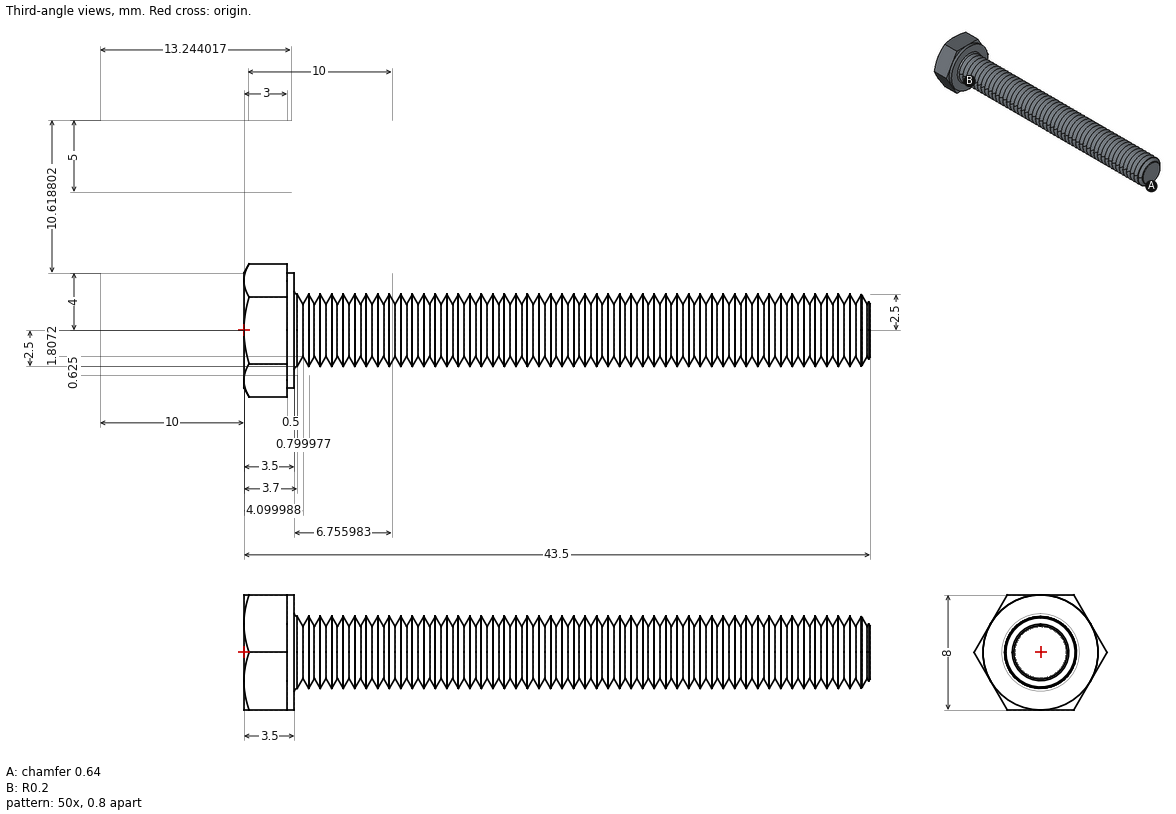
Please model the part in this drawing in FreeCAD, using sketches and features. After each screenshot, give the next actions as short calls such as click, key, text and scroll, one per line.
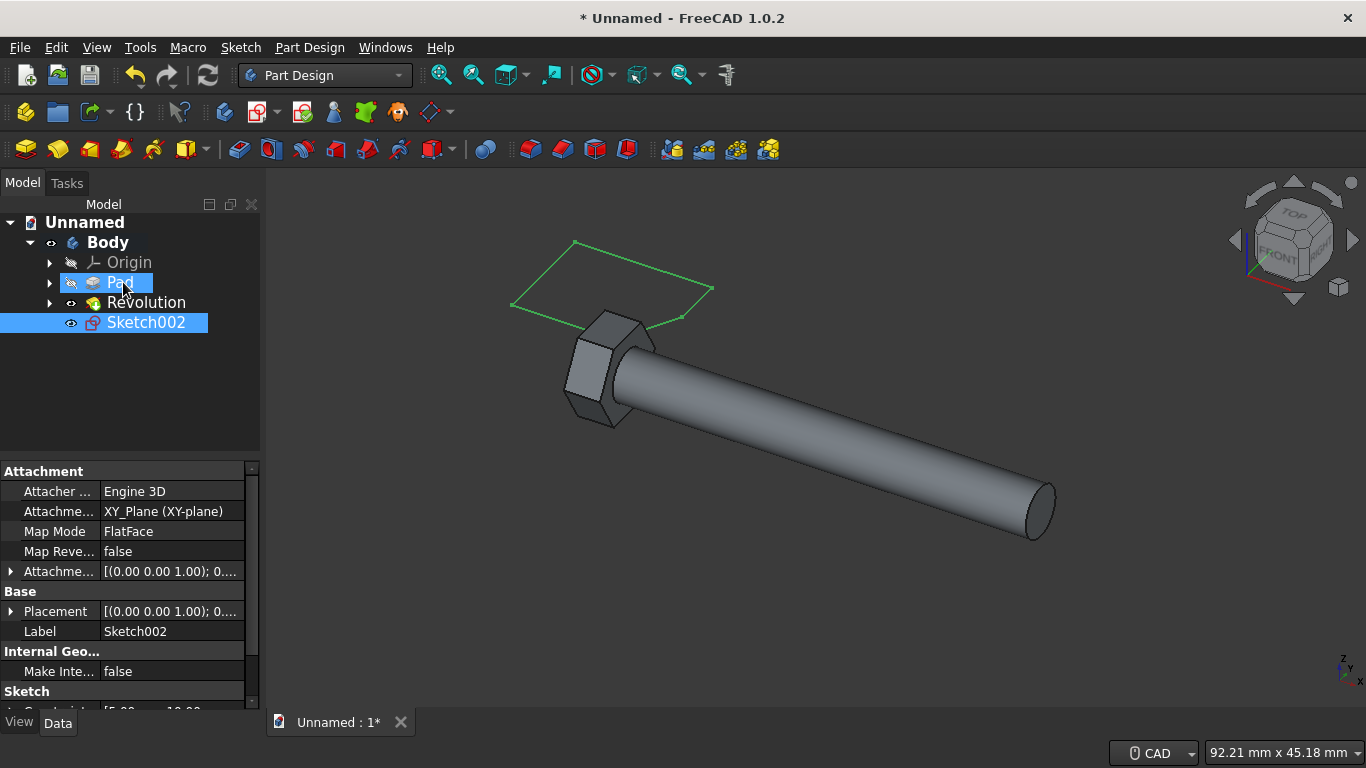
click(304, 150)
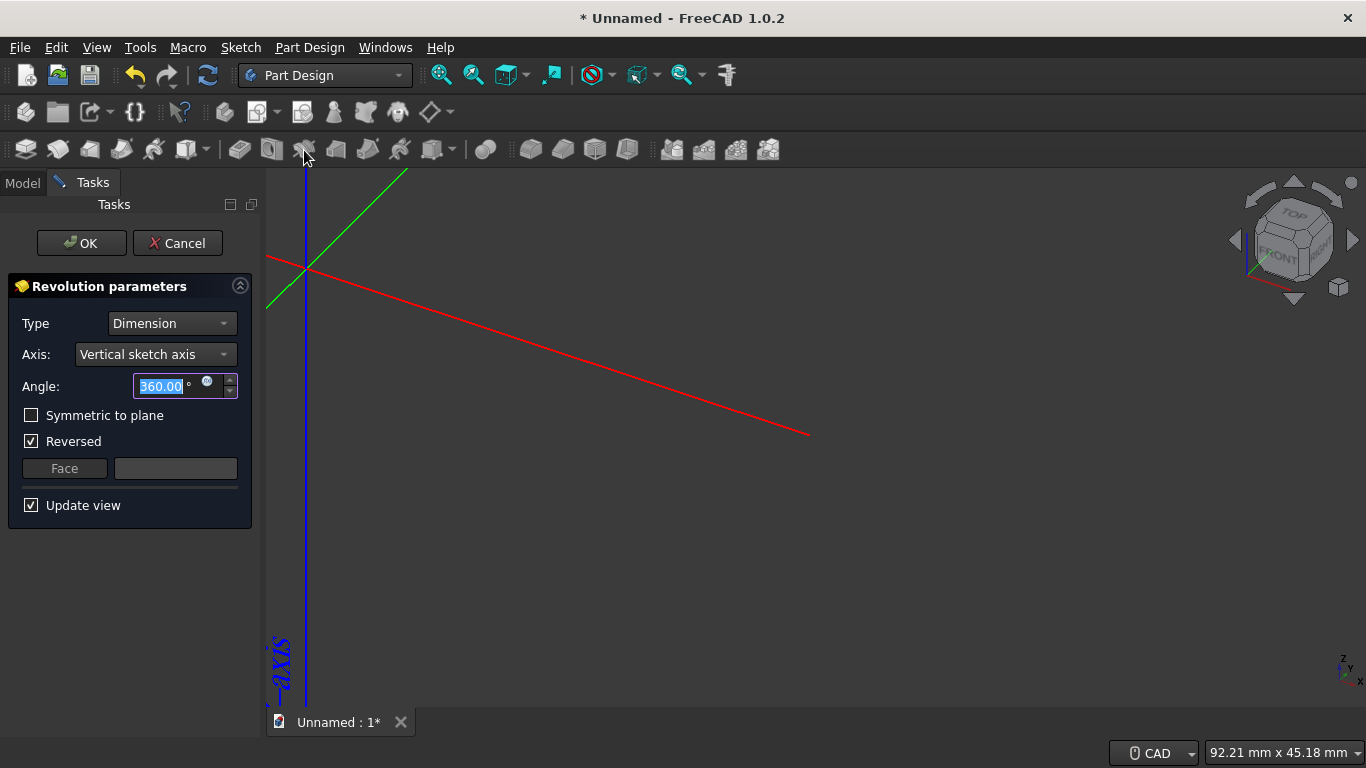
click(156, 354)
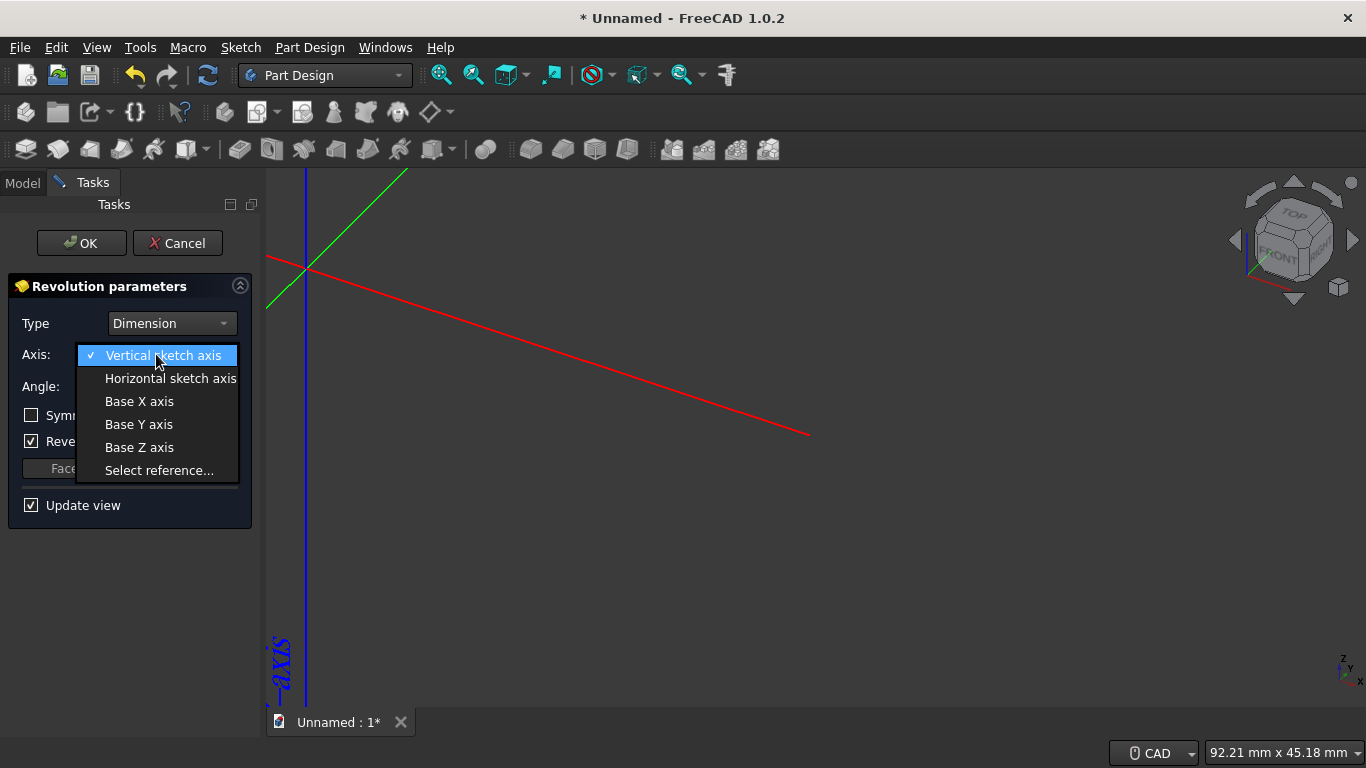
click(156, 378)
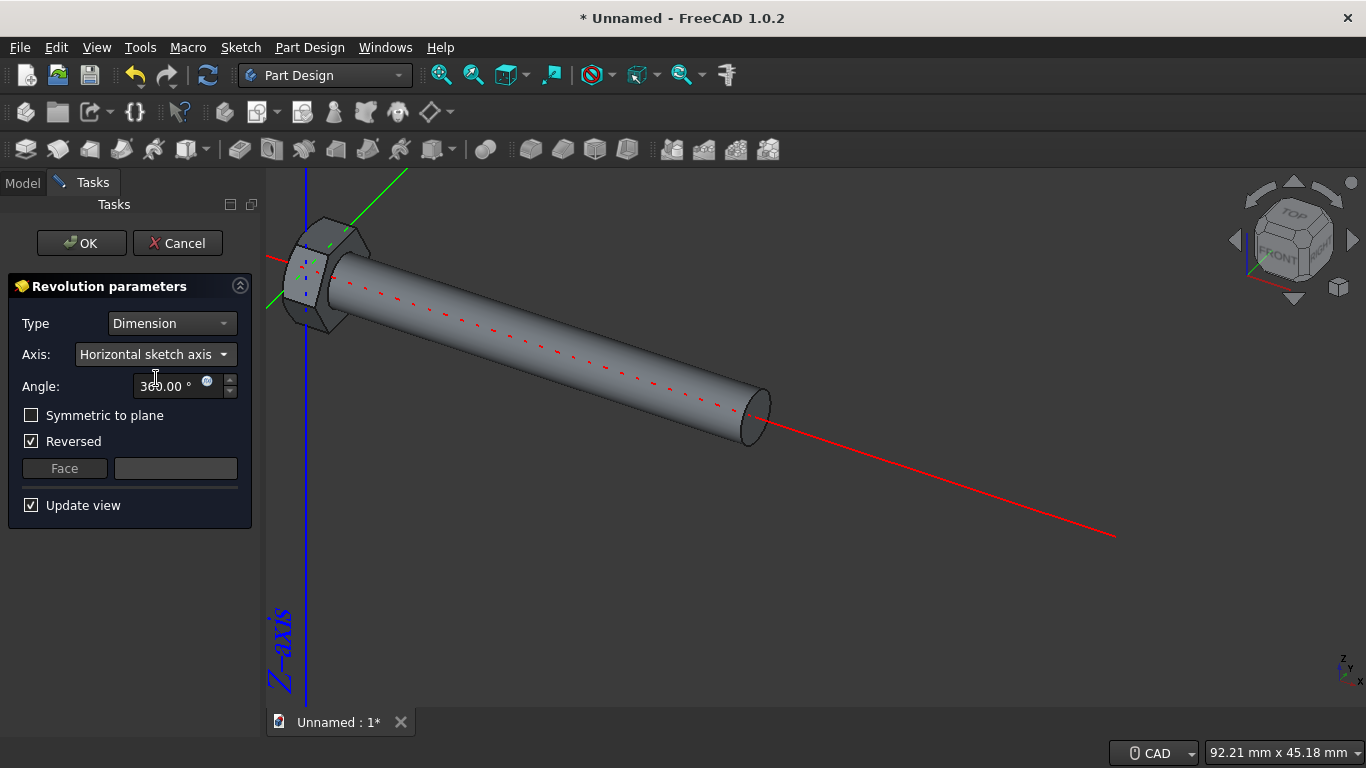
click(82, 243)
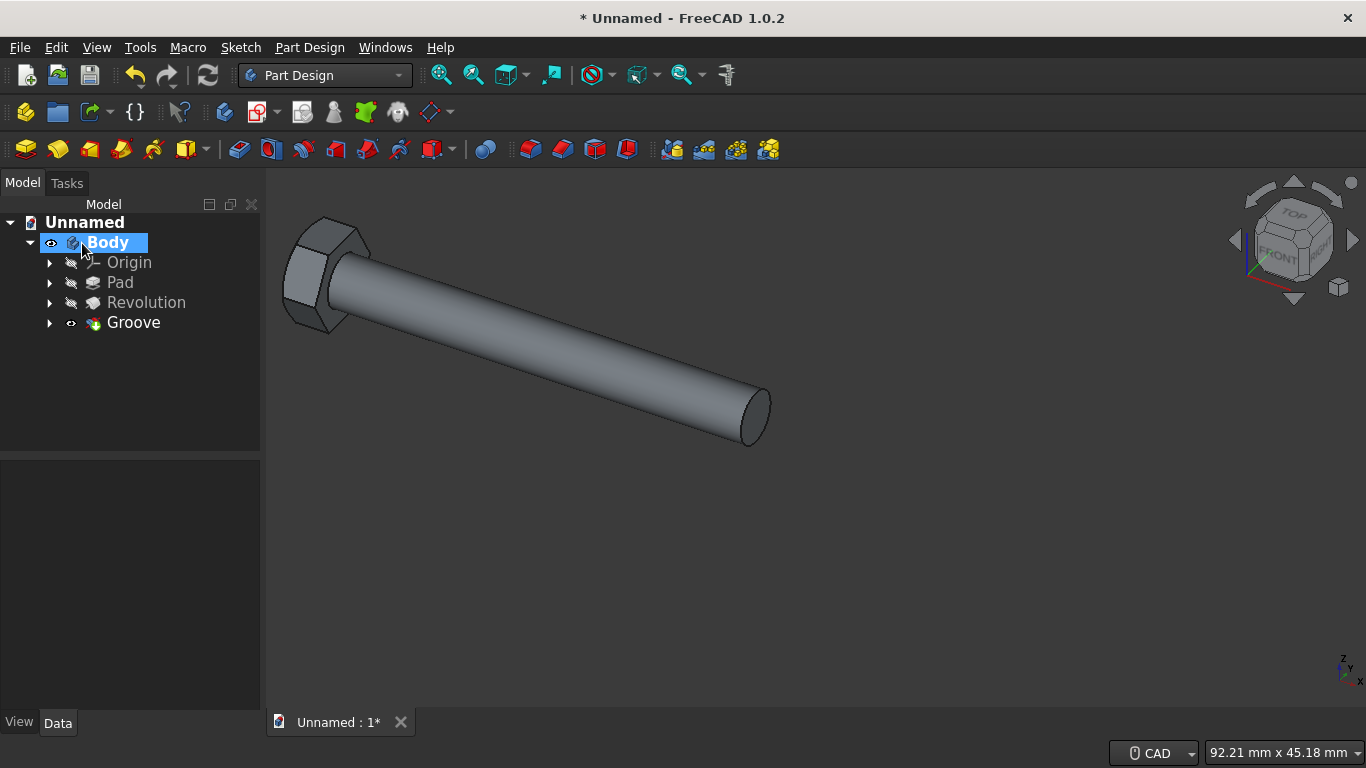
click(258, 112)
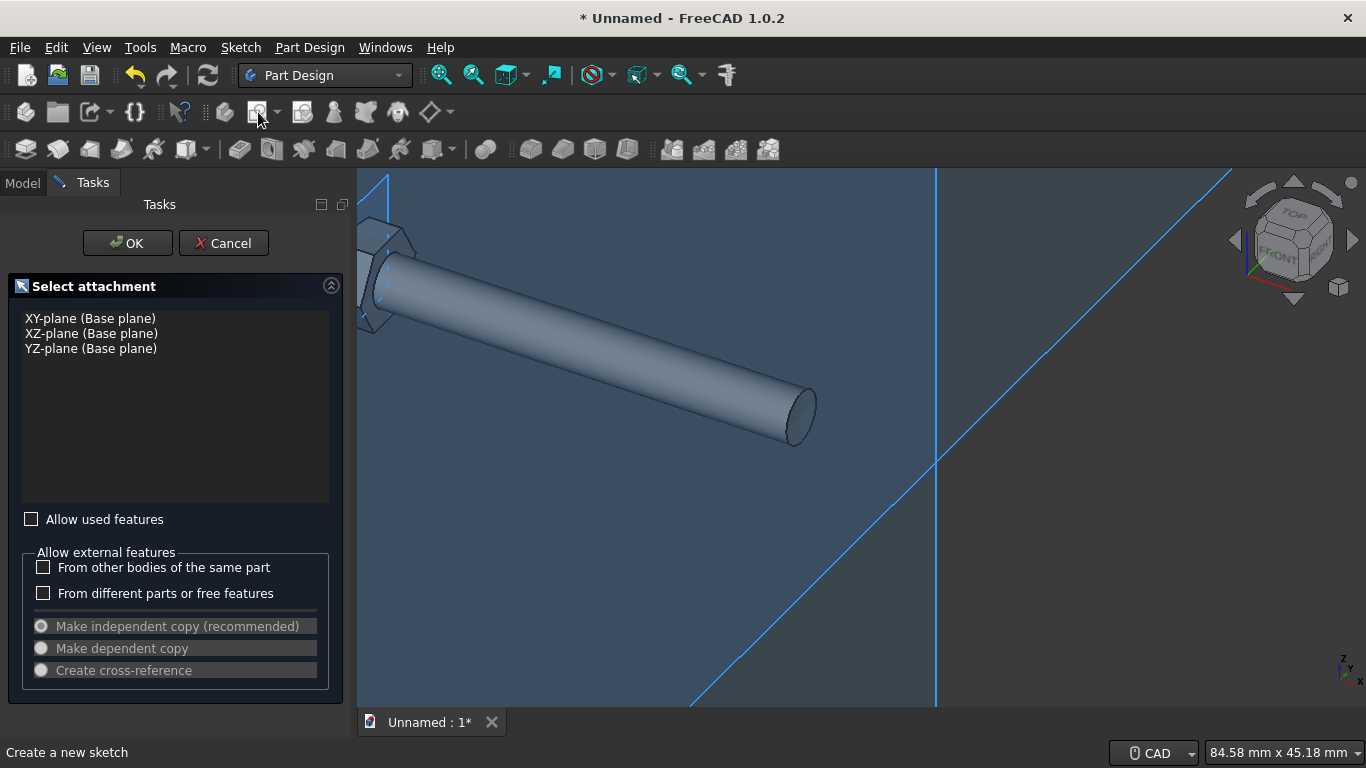
click(82, 318)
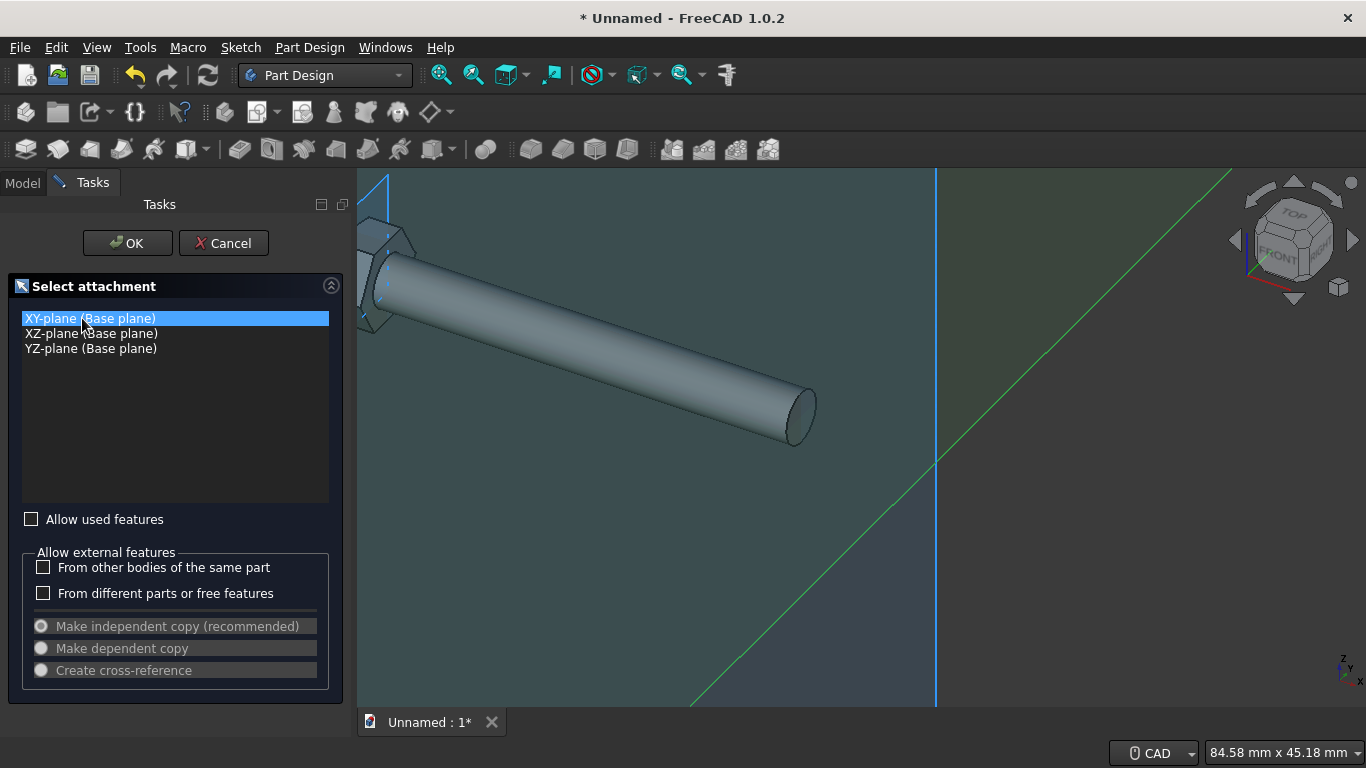
click(128, 243)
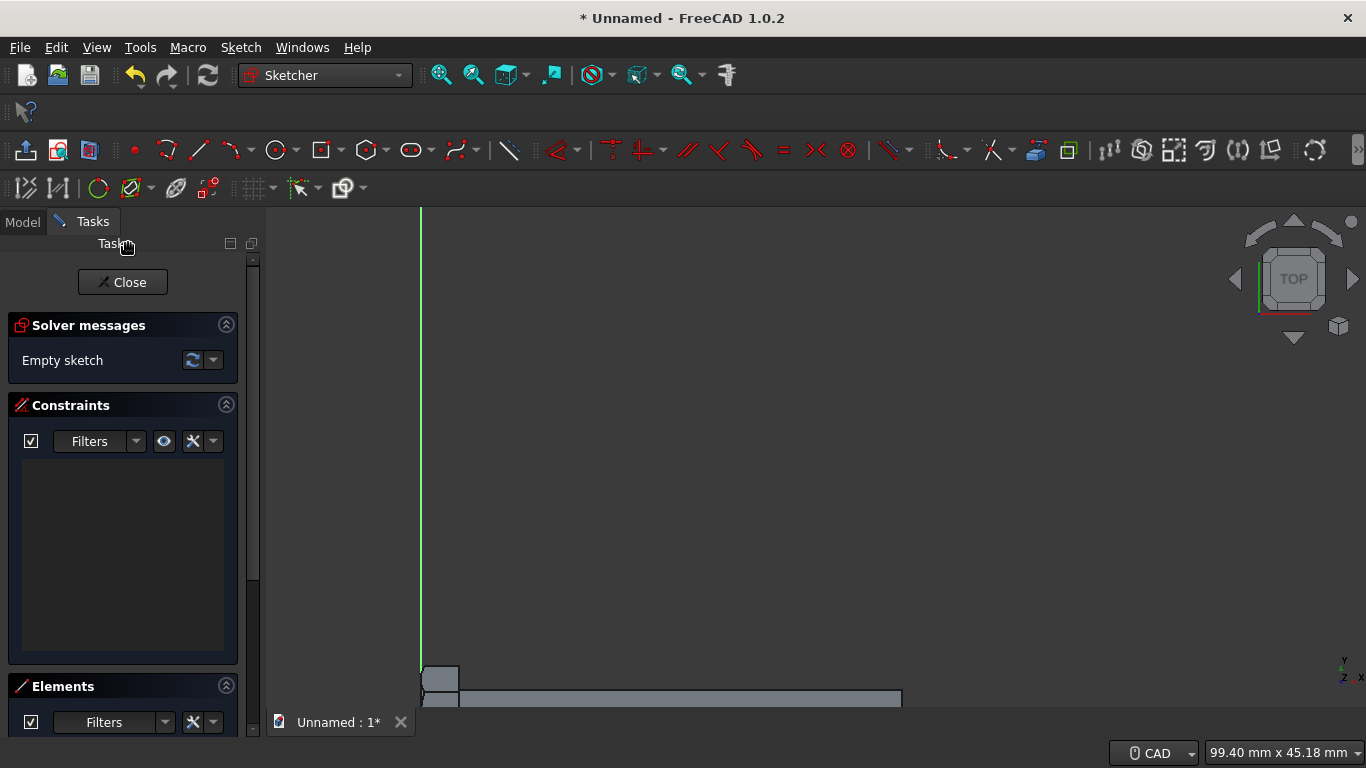
click(90, 150)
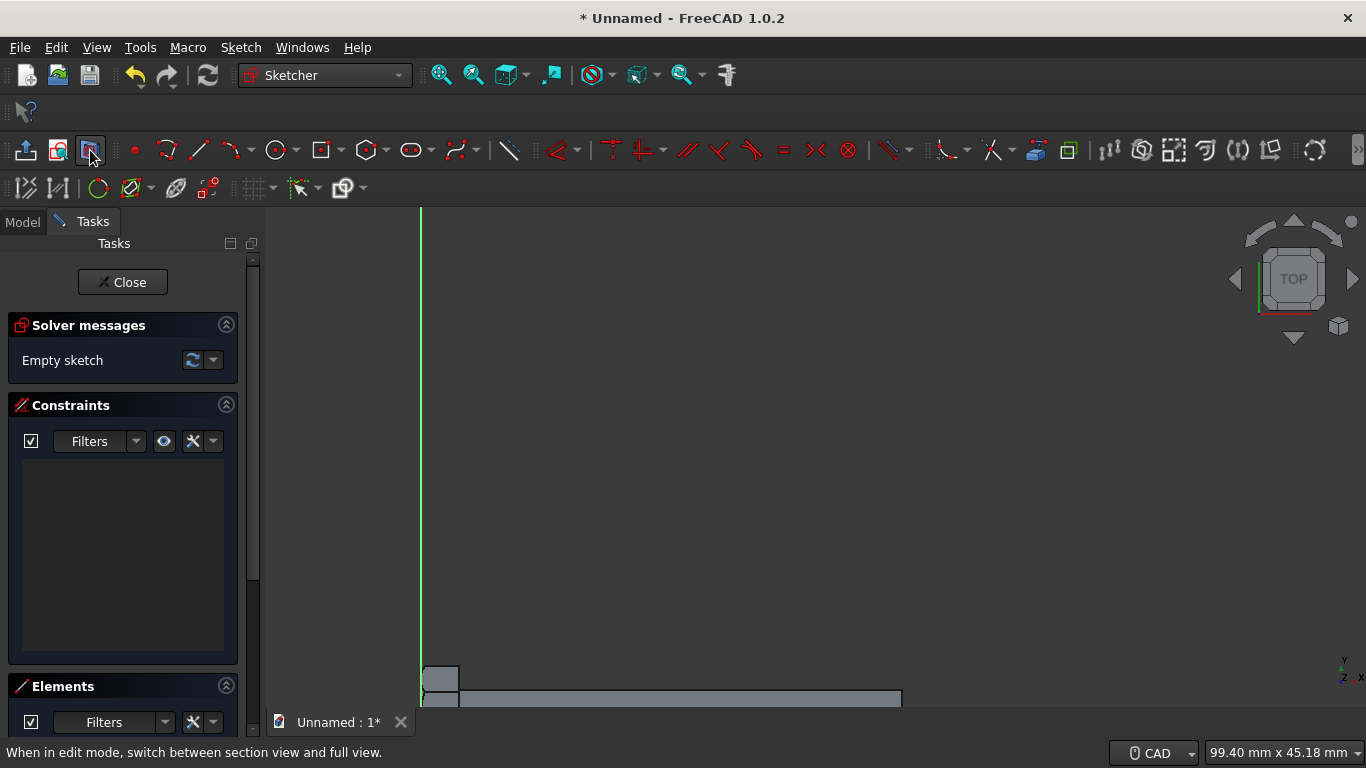
scroll(748, 457, down, 5)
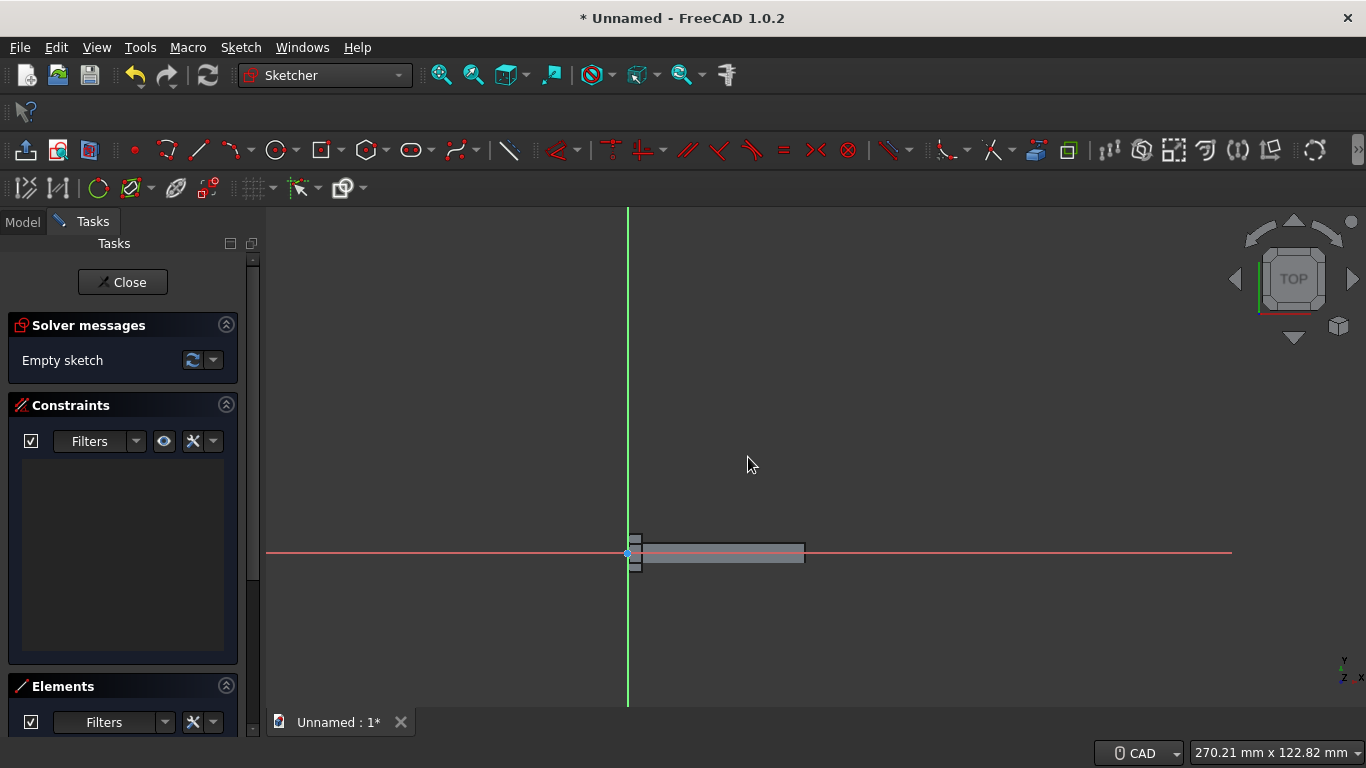
scroll(624, 540, up, 8)